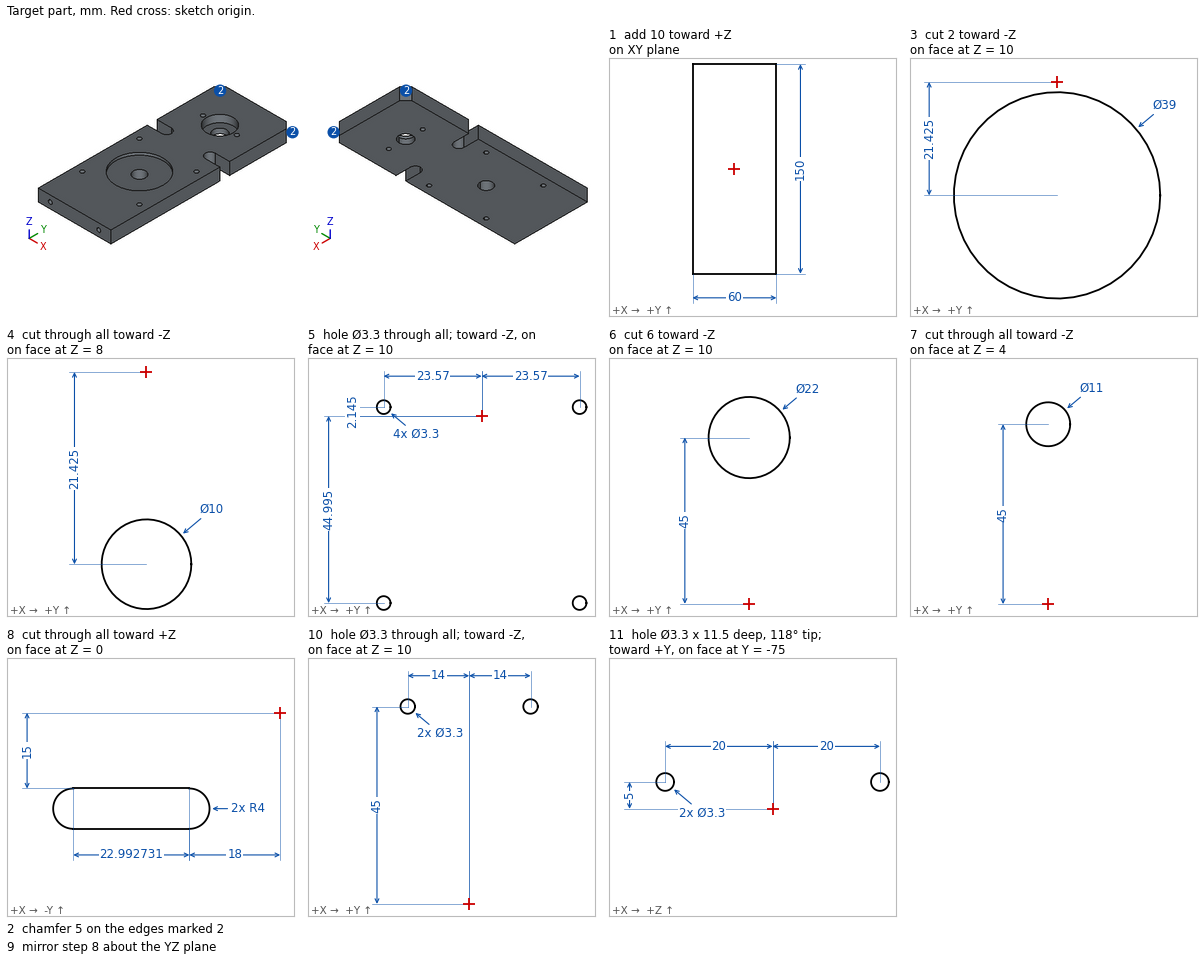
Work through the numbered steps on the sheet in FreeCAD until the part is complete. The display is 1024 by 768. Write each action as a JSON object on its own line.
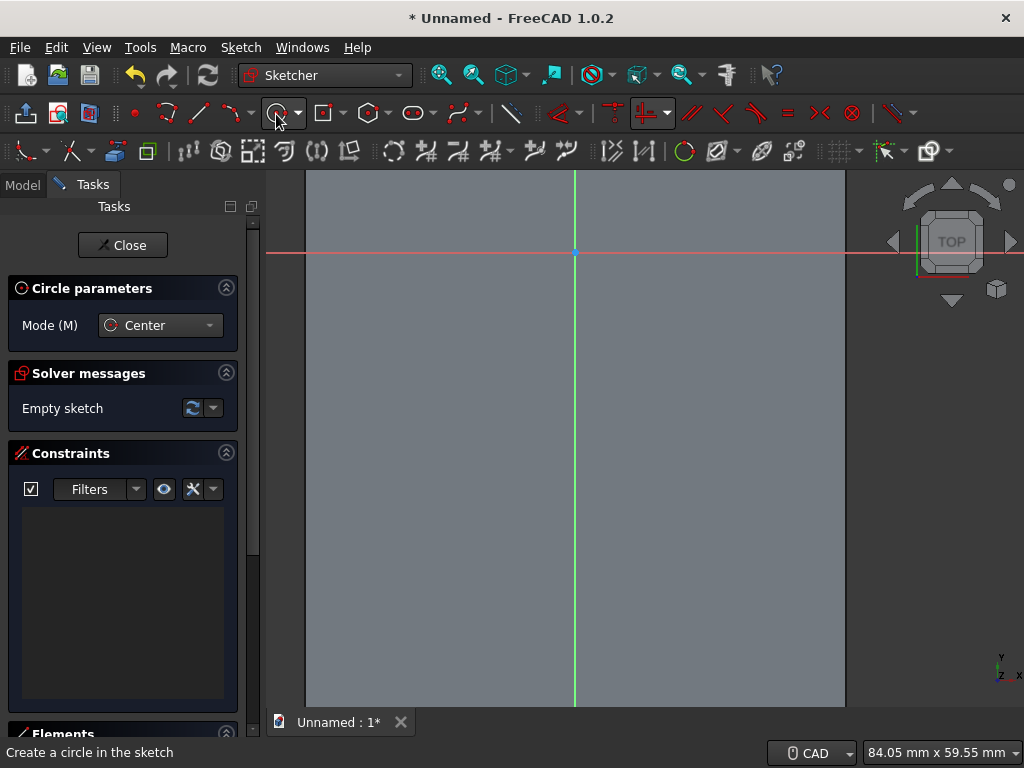
{"action": "left_click", "coordinate": [575, 446]}
{"action": "left_click", "coordinate": [700, 321]}
{"action": "key", "text": "Escape"}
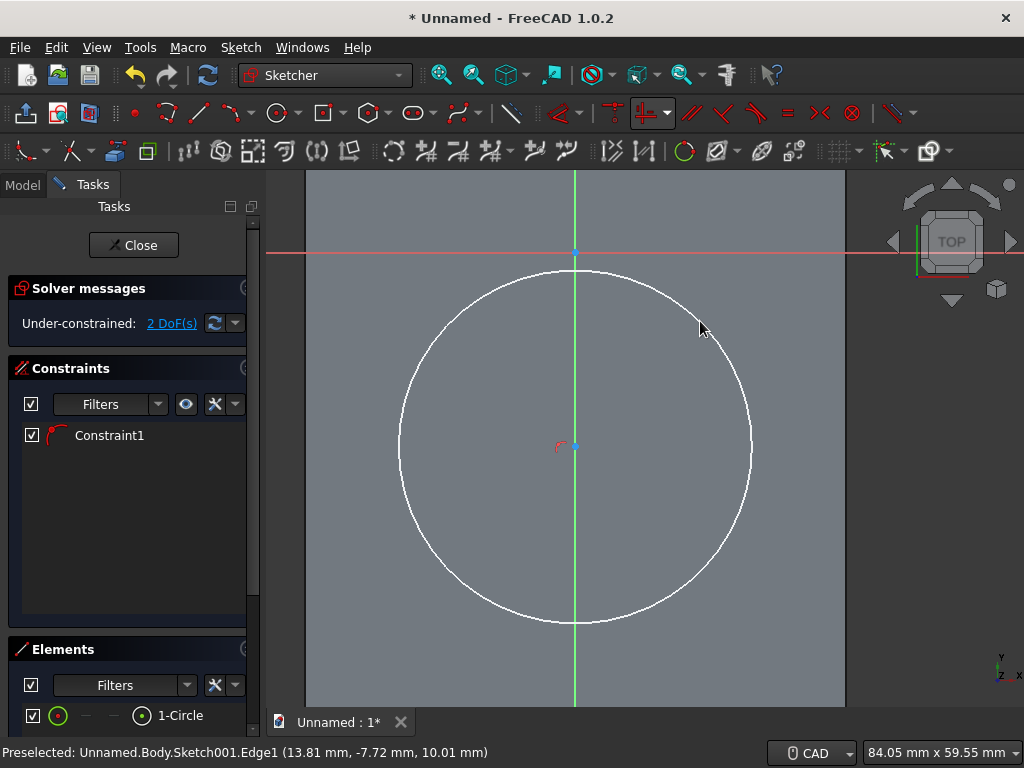
{"action": "left_click", "coordinate": [558, 114]}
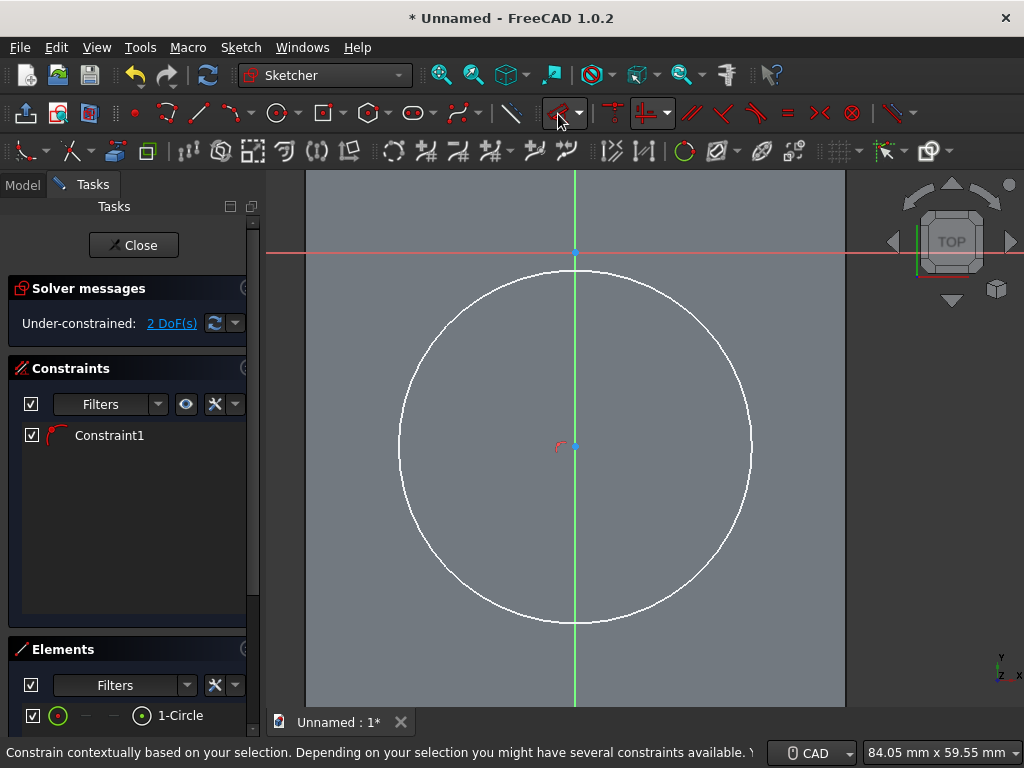
{"action": "left_click", "coordinate": [700, 322]}
{"action": "left_click", "coordinate": [723, 299]}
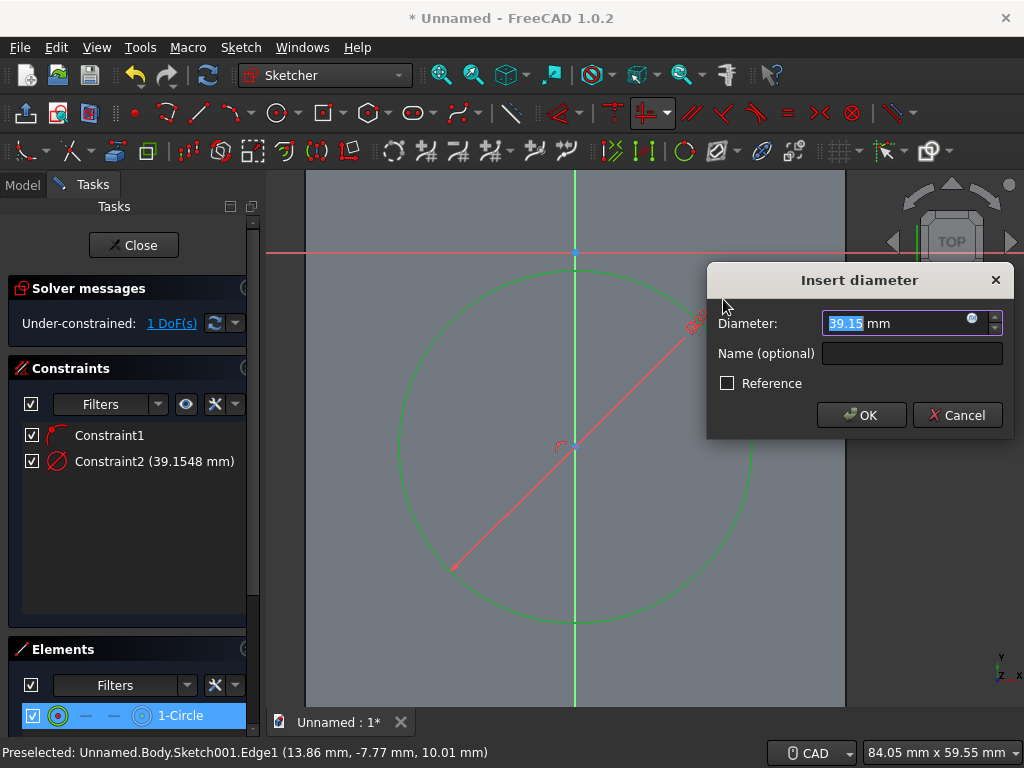
{"action": "type", "text": "39"}
{"action": "key", "text": "Return"}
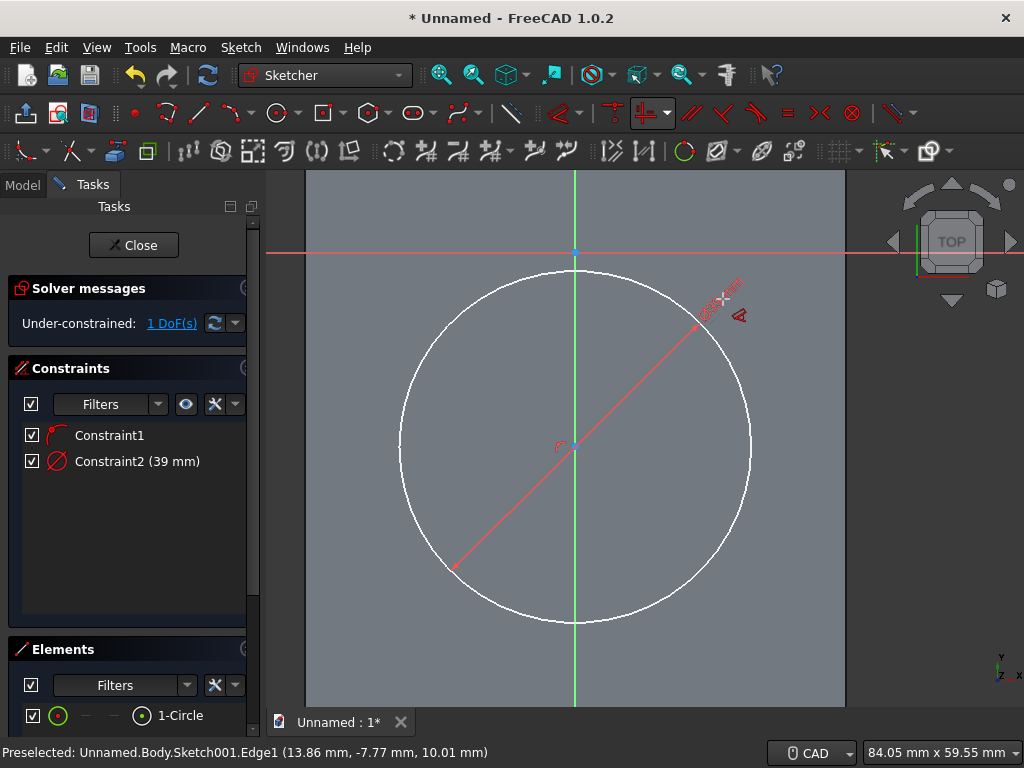
{"action": "left_click", "coordinate": [575, 447]}
{"action": "left_click", "coordinate": [609, 350]}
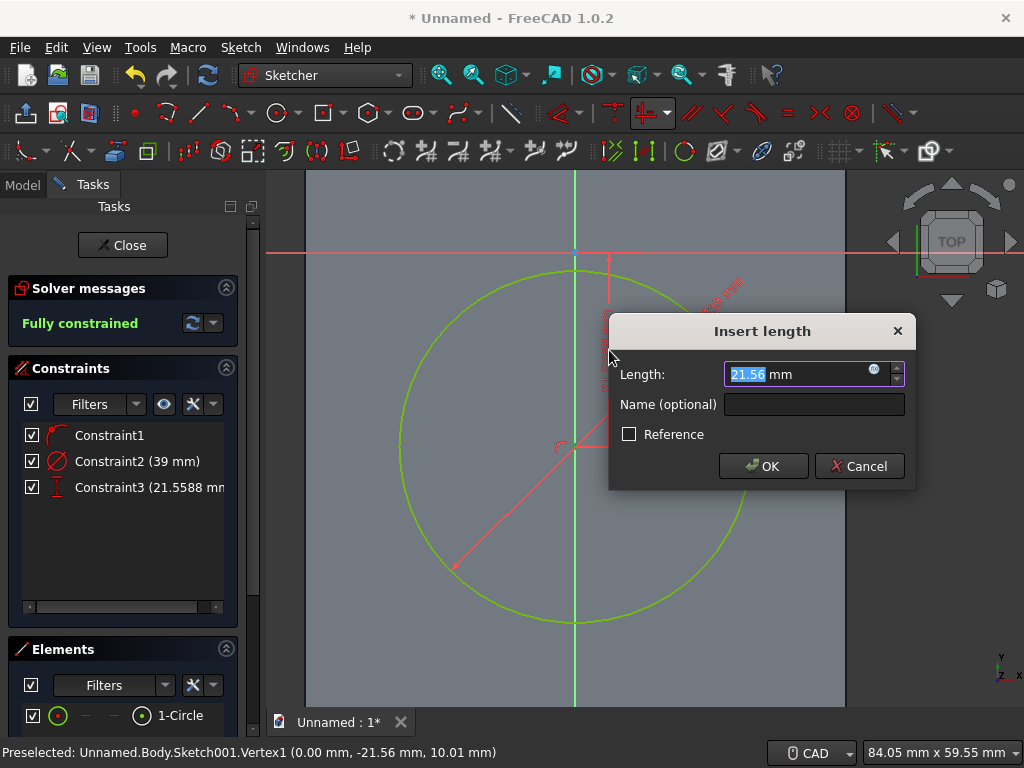
{"action": "type", "text": "21.425"}
{"action": "key", "text": "Return"}
{"action": "key", "text": "Escape"}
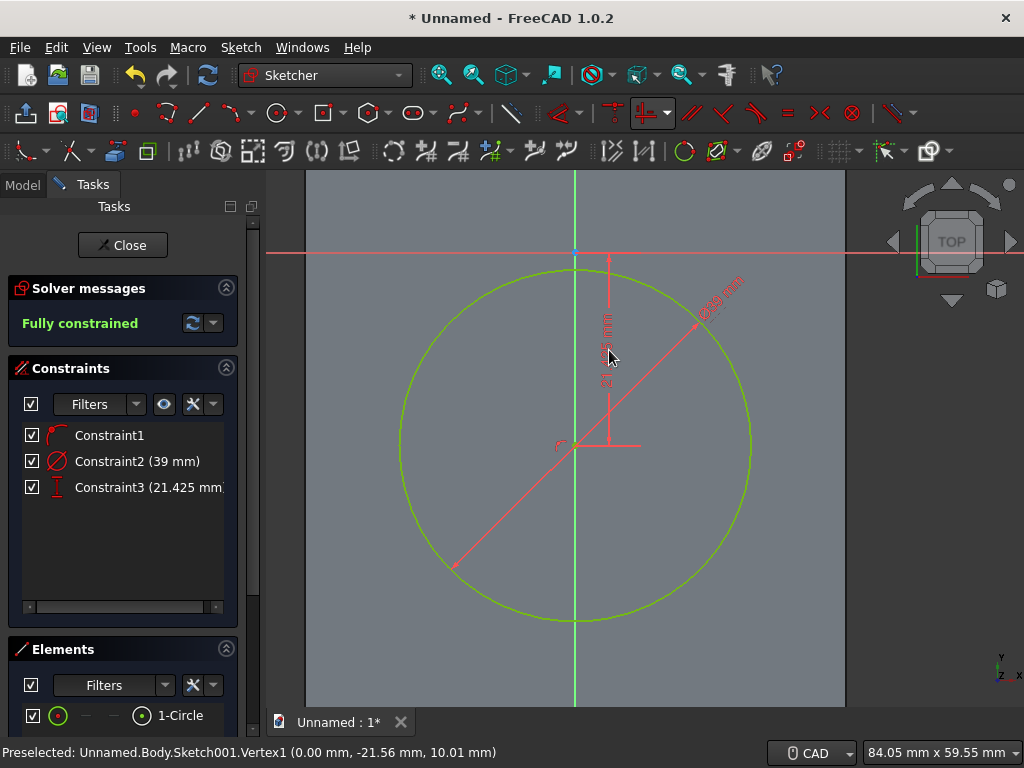
{"action": "left_click", "coordinate": [123, 245]}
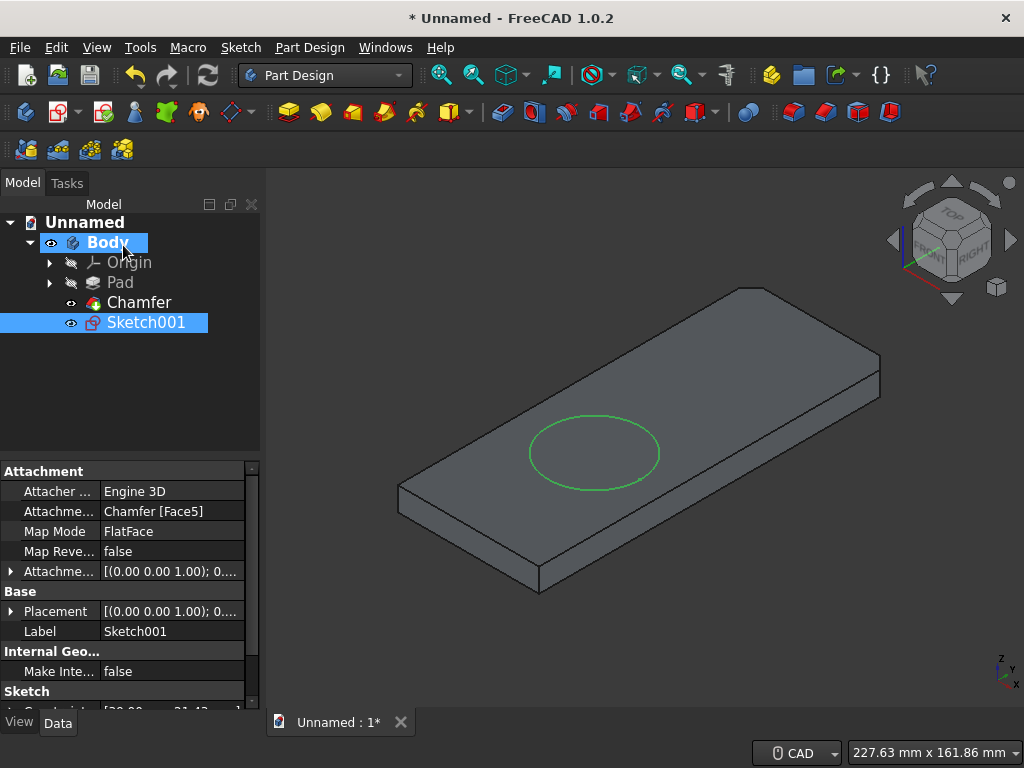
{"action": "left_click", "coordinate": [504, 112]}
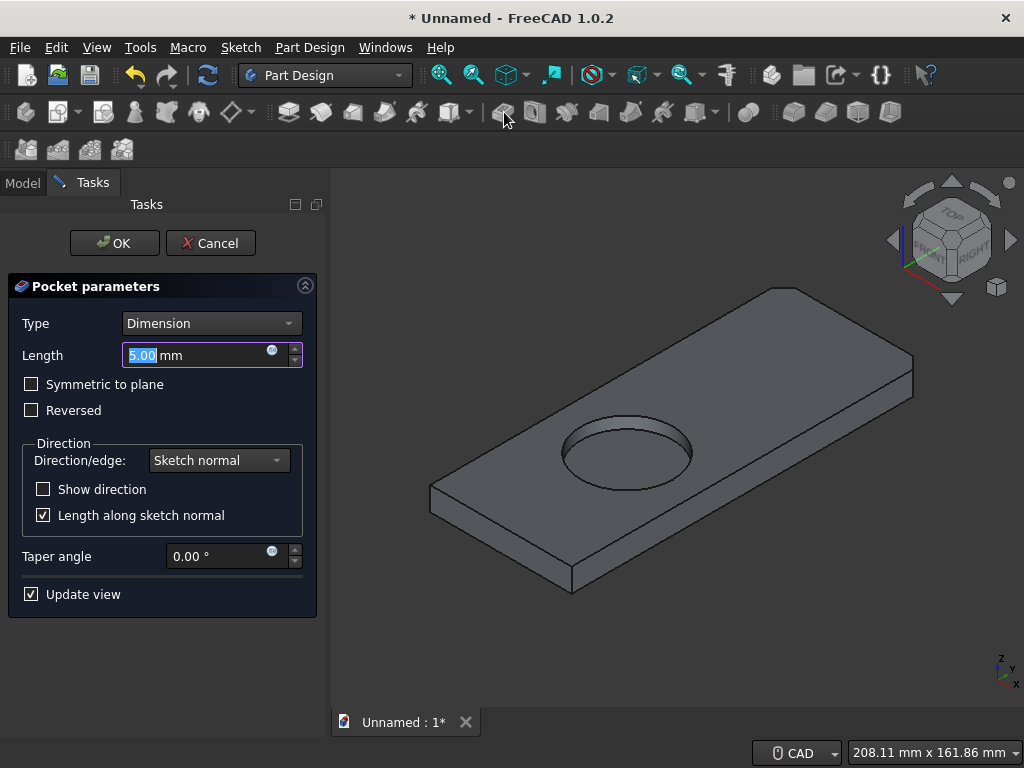
{"action": "type", "text": "2"}
{"action": "key", "text": "Tab"}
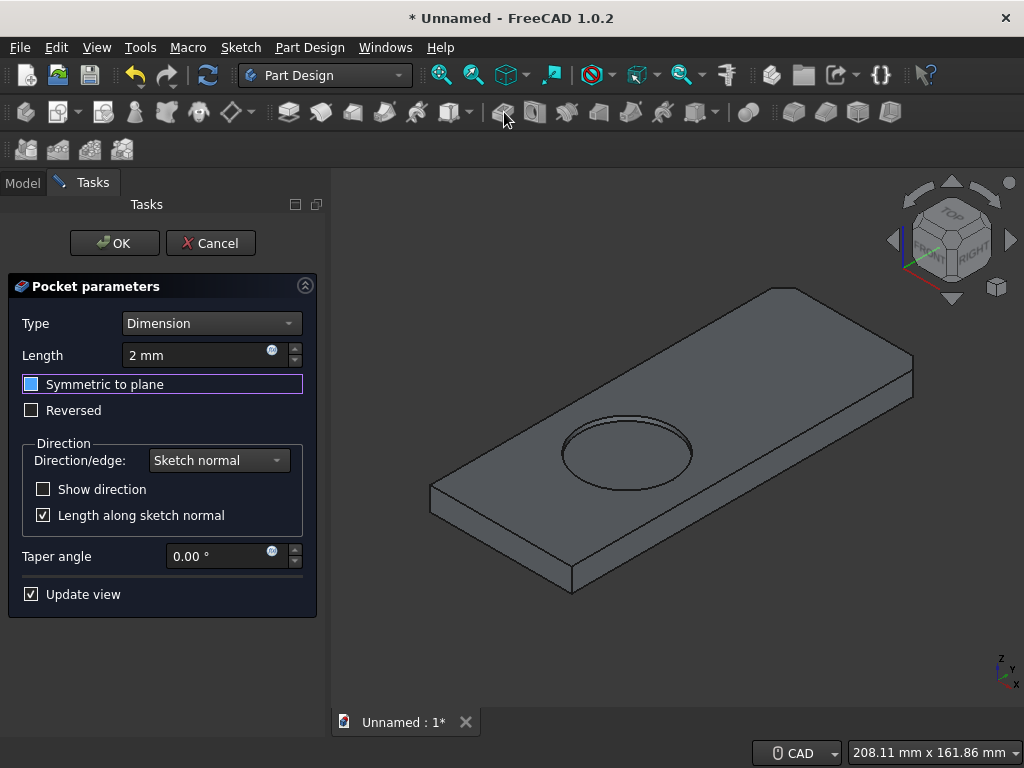
{"action": "left_click", "coordinate": [115, 243]}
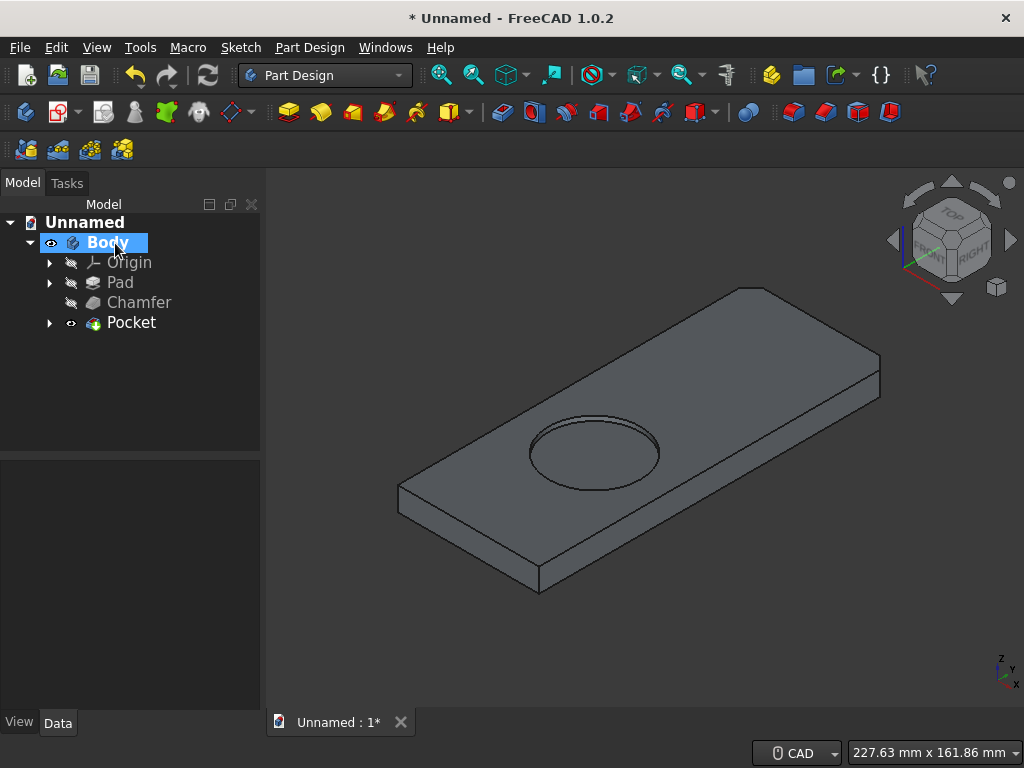
{"action": "left_click", "coordinate": [595, 457]}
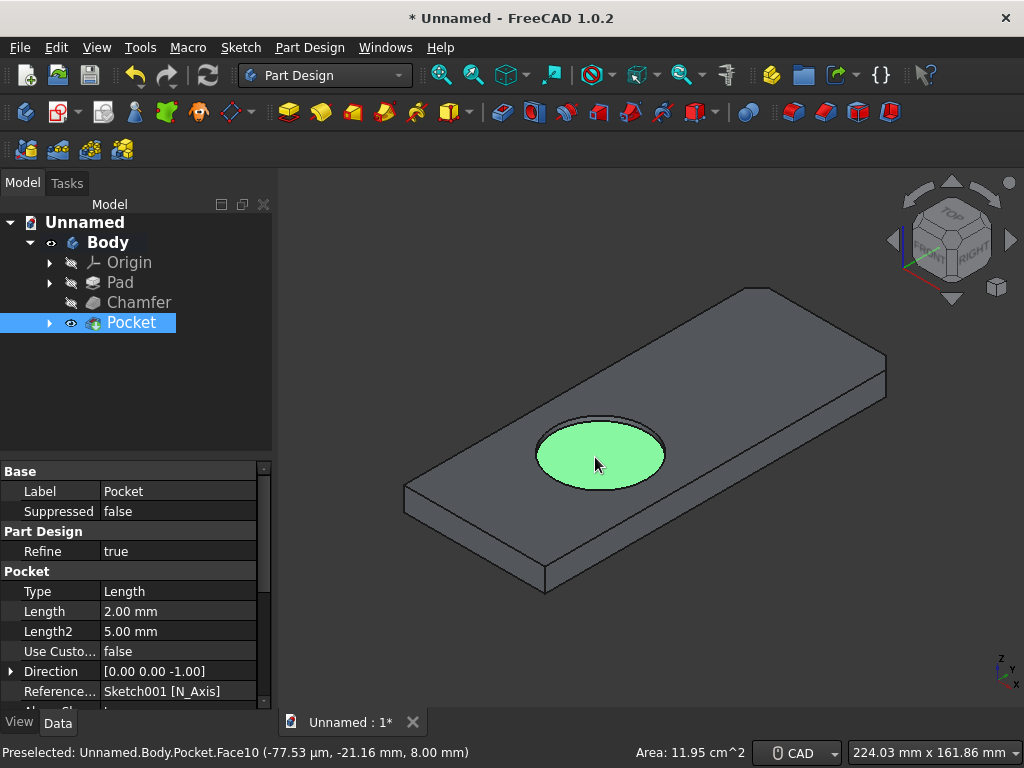
{"action": "left_click", "coordinate": [58, 112]}